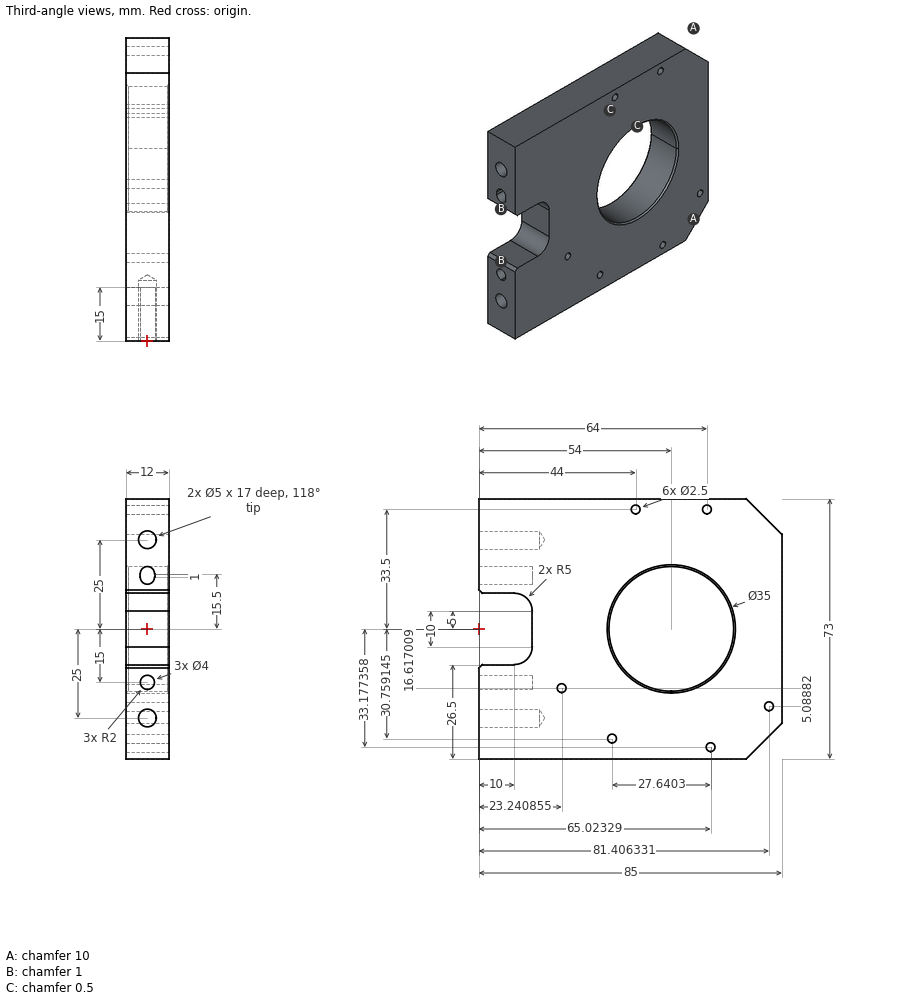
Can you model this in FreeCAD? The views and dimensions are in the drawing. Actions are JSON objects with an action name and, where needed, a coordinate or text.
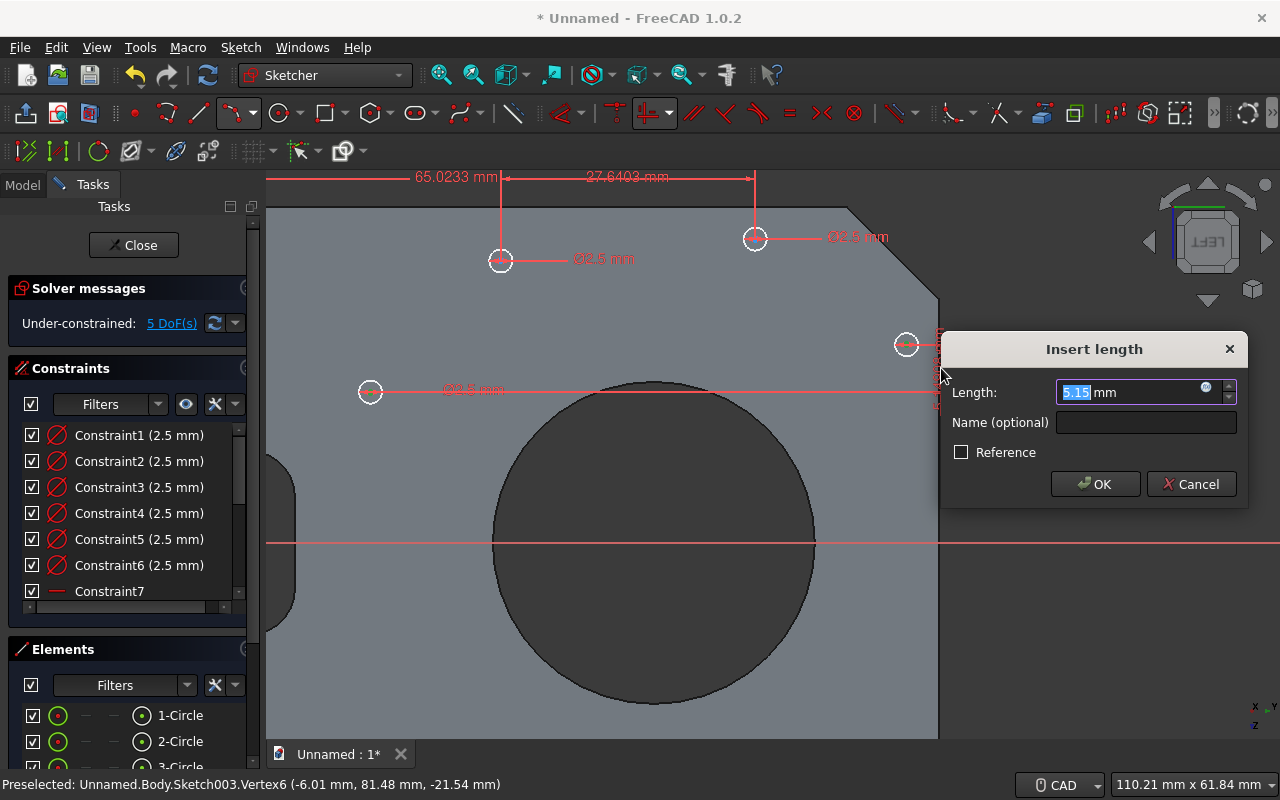
{"action": "type", "text": "5.08882"}
{"action": "key", "text": "Return"}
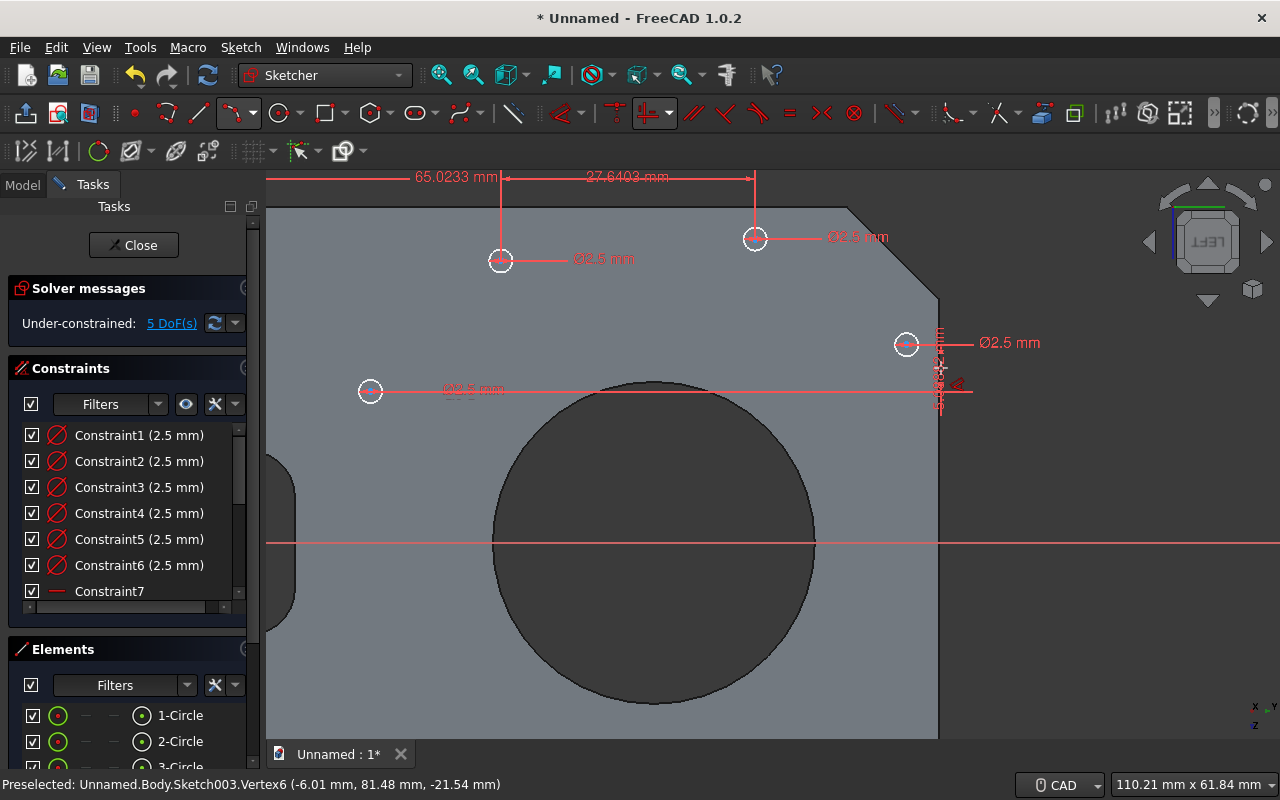
{"action": "left_click", "coordinate": [371, 392]}
{"action": "left_click", "coordinate": [332, 358]}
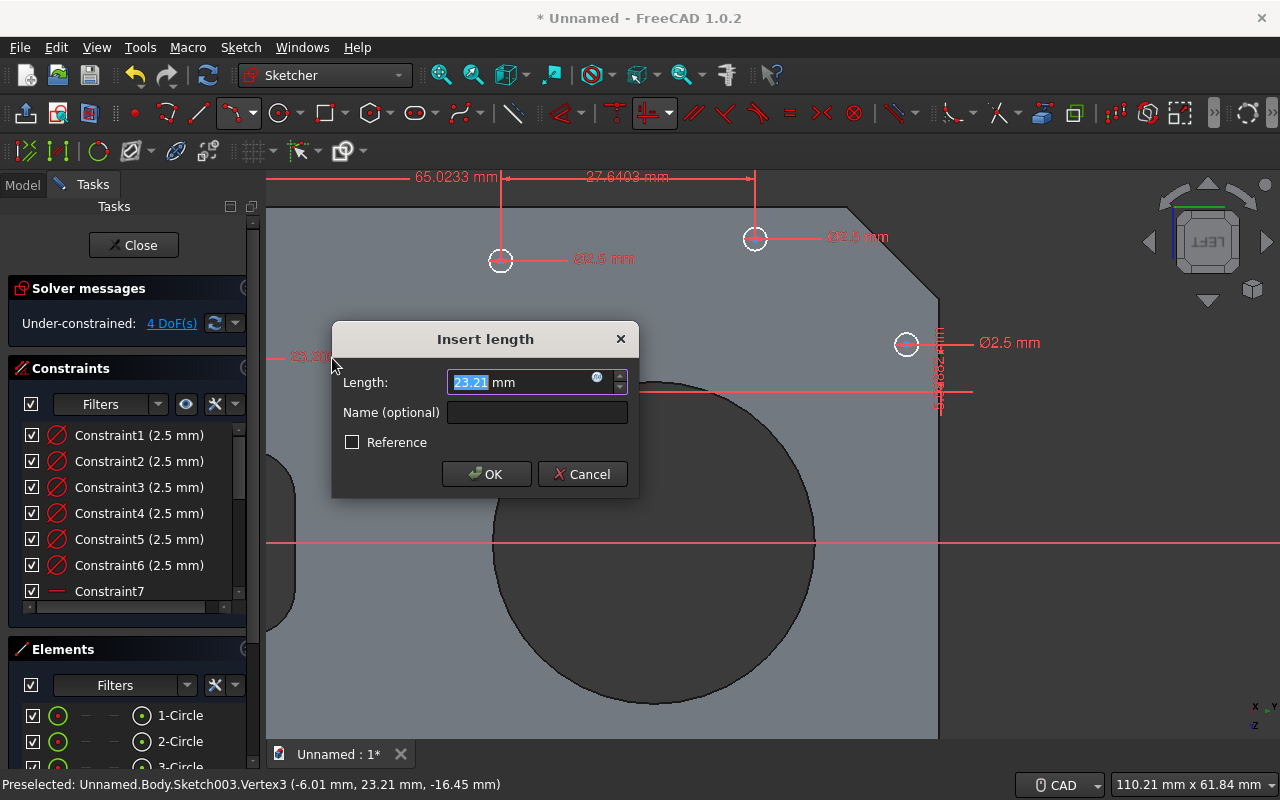
{"action": "type", "text": "23.240855"}
{"action": "key", "text": "Return"}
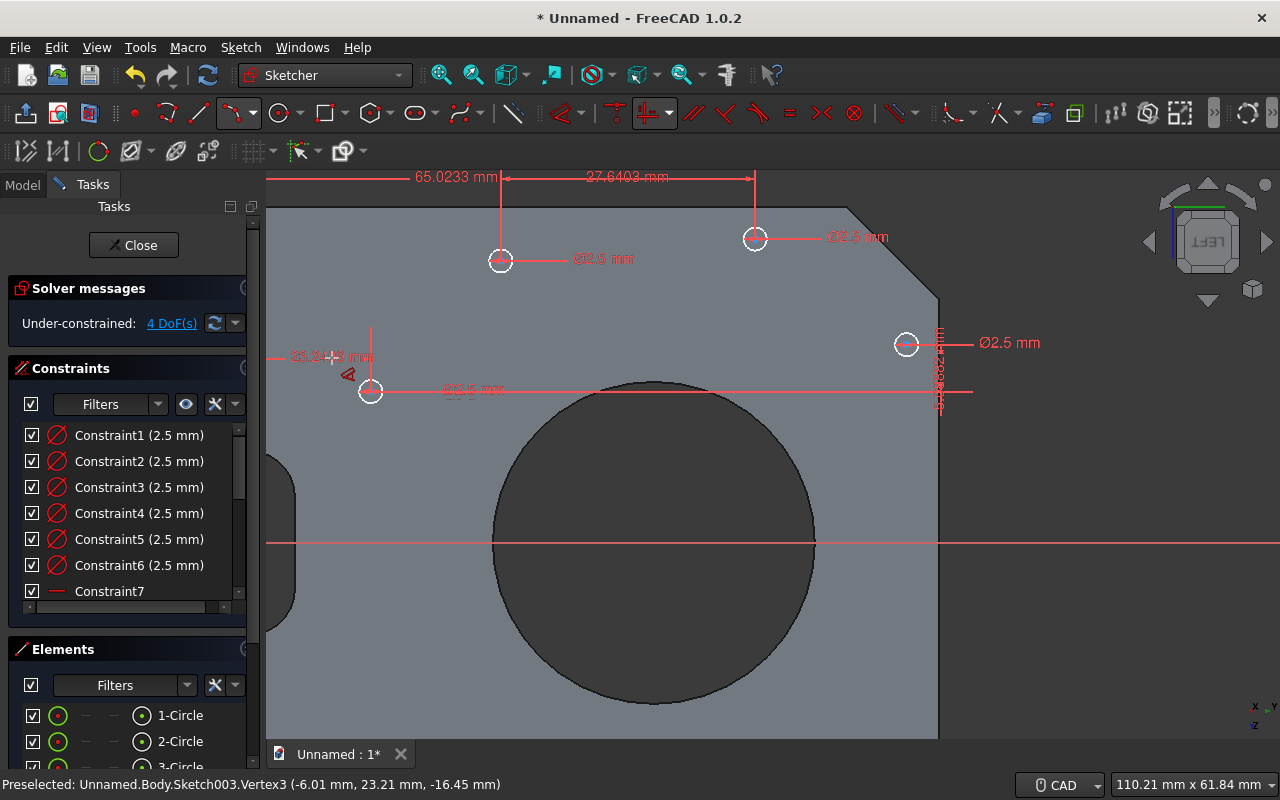
{"action": "left_click", "coordinate": [371, 392]}
{"action": "left_click", "coordinate": [405, 467]}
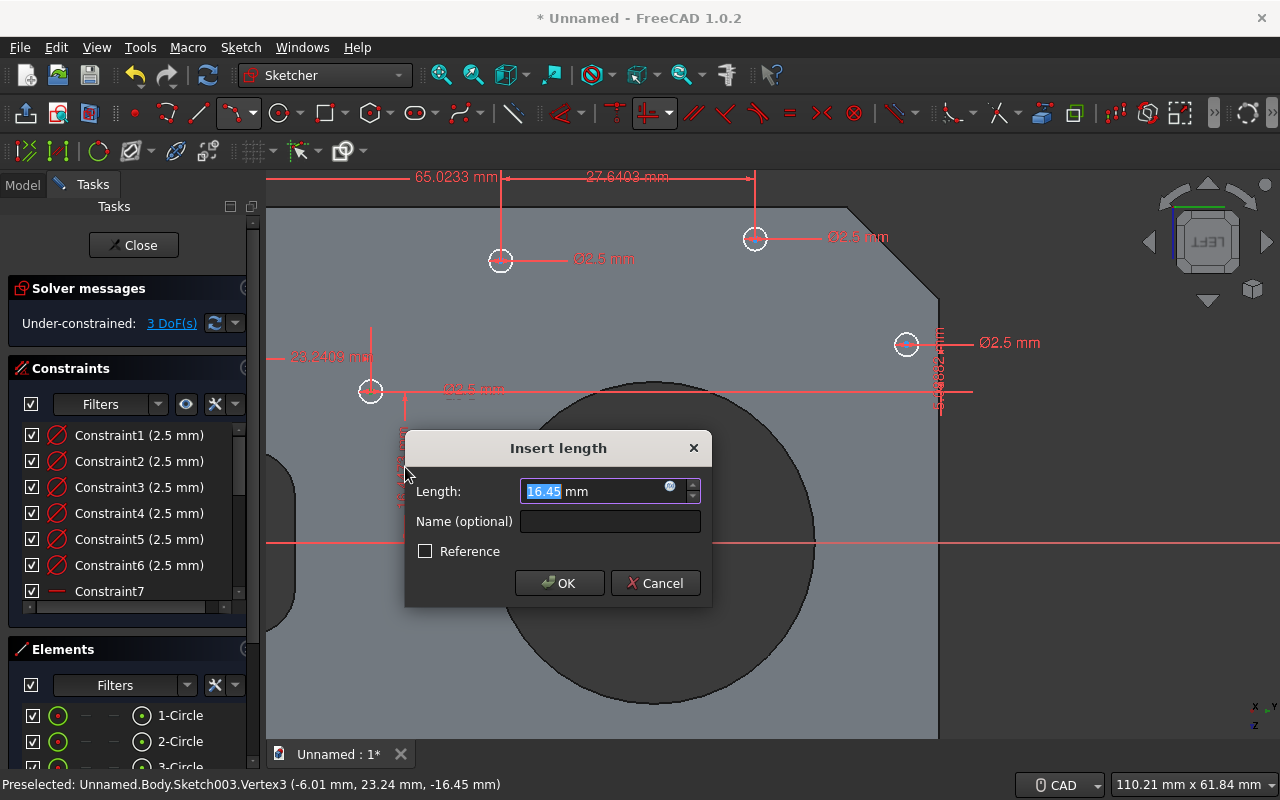
{"action": "type", "text": "16.617009"}
{"action": "key", "text": "Return"}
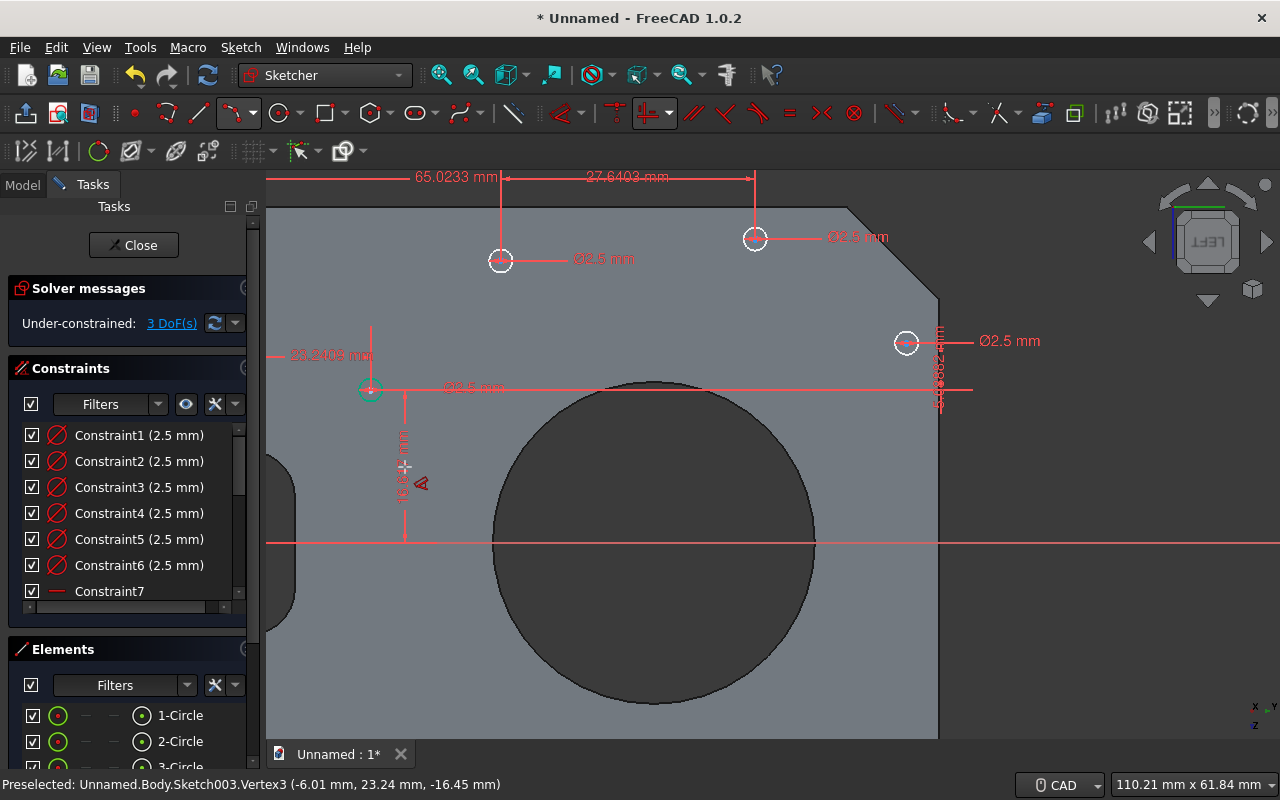
{"action": "left_click", "coordinate": [501, 261]}
{"action": "left_click", "coordinate": [535, 402]}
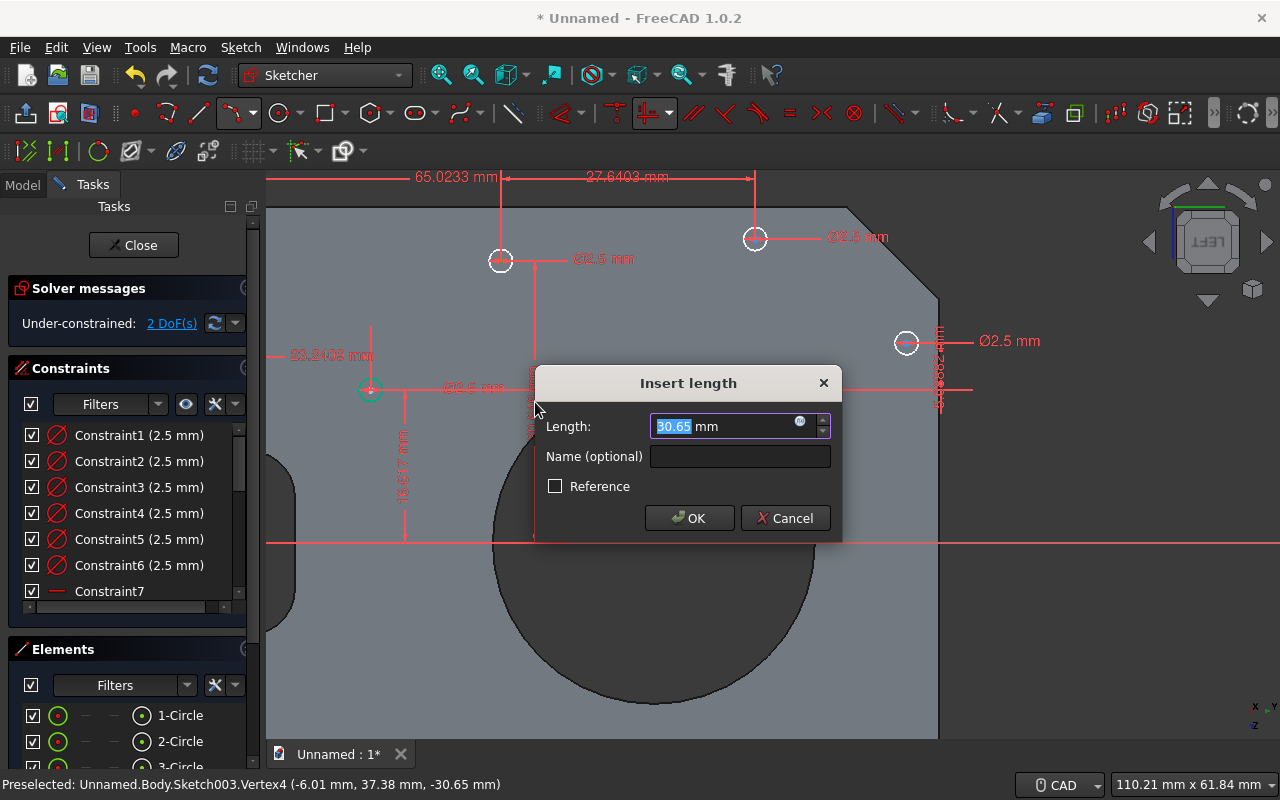
{"action": "type", "text": "30.759145"}
{"action": "key", "text": "Return"}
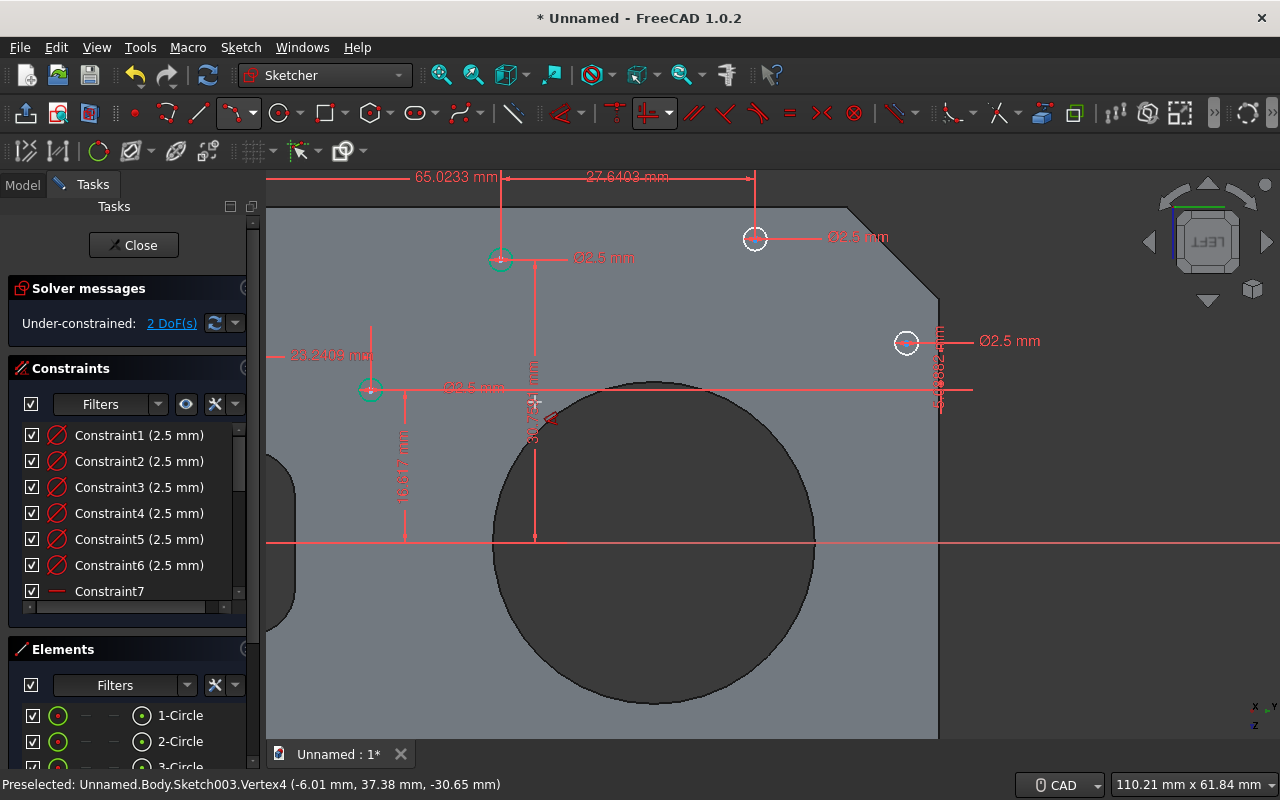
{"action": "left_click", "coordinate": [755, 239]}
{"action": "left_click", "coordinate": [789, 391]}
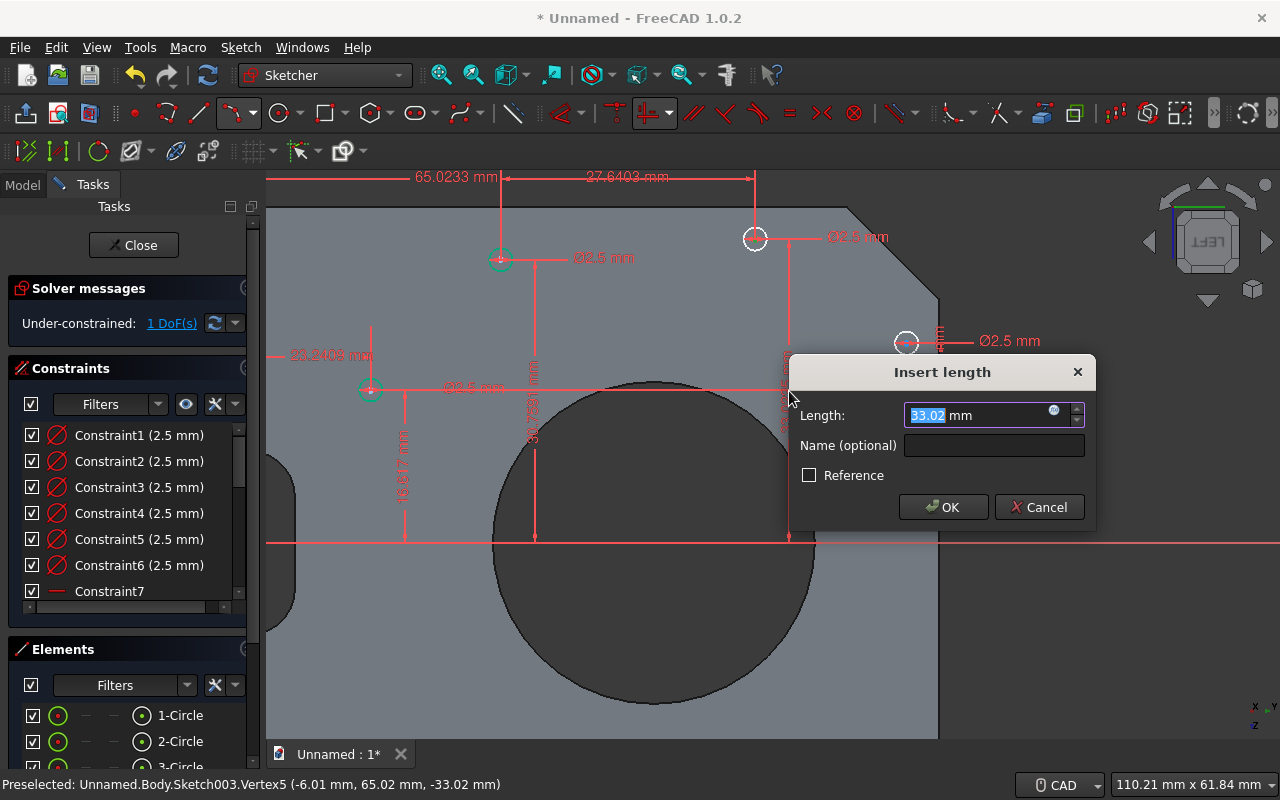
{"action": "type", "text": "33.177358"}
{"action": "key", "text": "Return"}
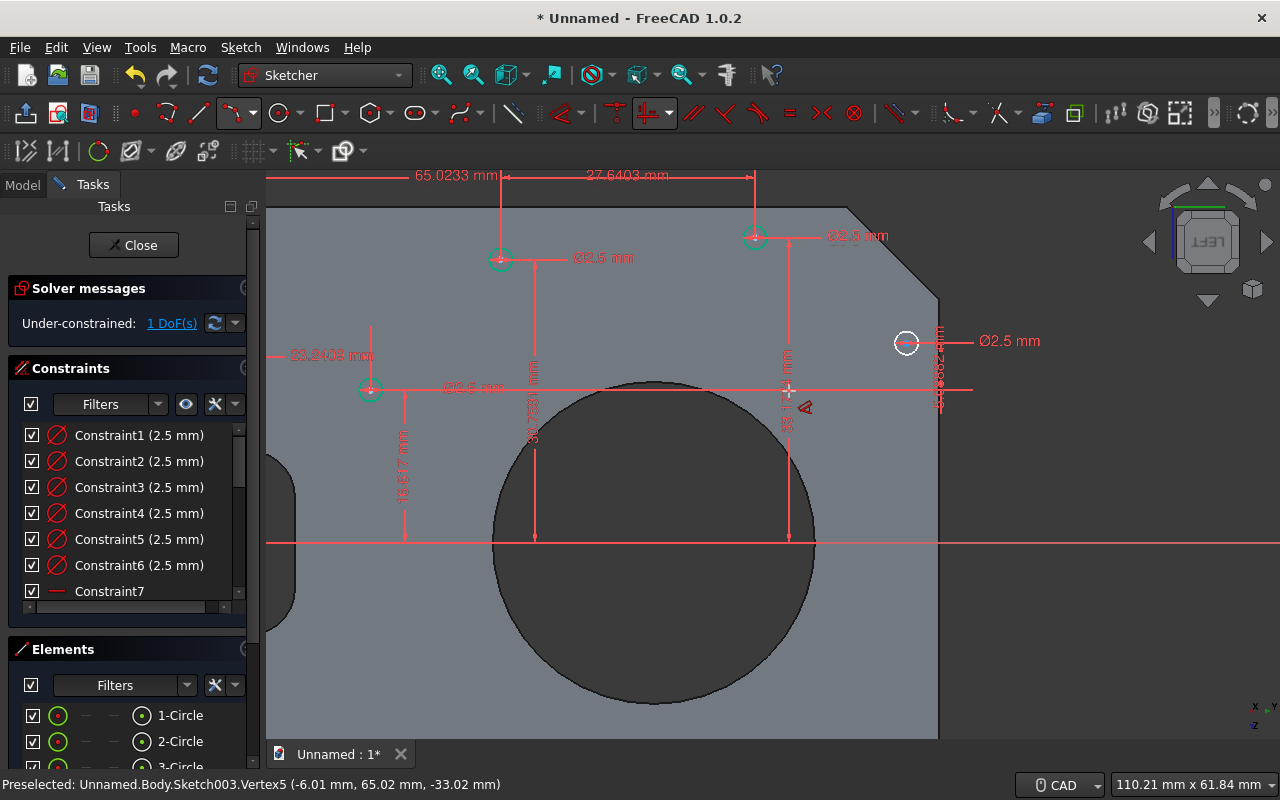
{"action": "left_click", "coordinate": [907, 343]}
{"action": "left_click", "coordinate": [600, 309]}